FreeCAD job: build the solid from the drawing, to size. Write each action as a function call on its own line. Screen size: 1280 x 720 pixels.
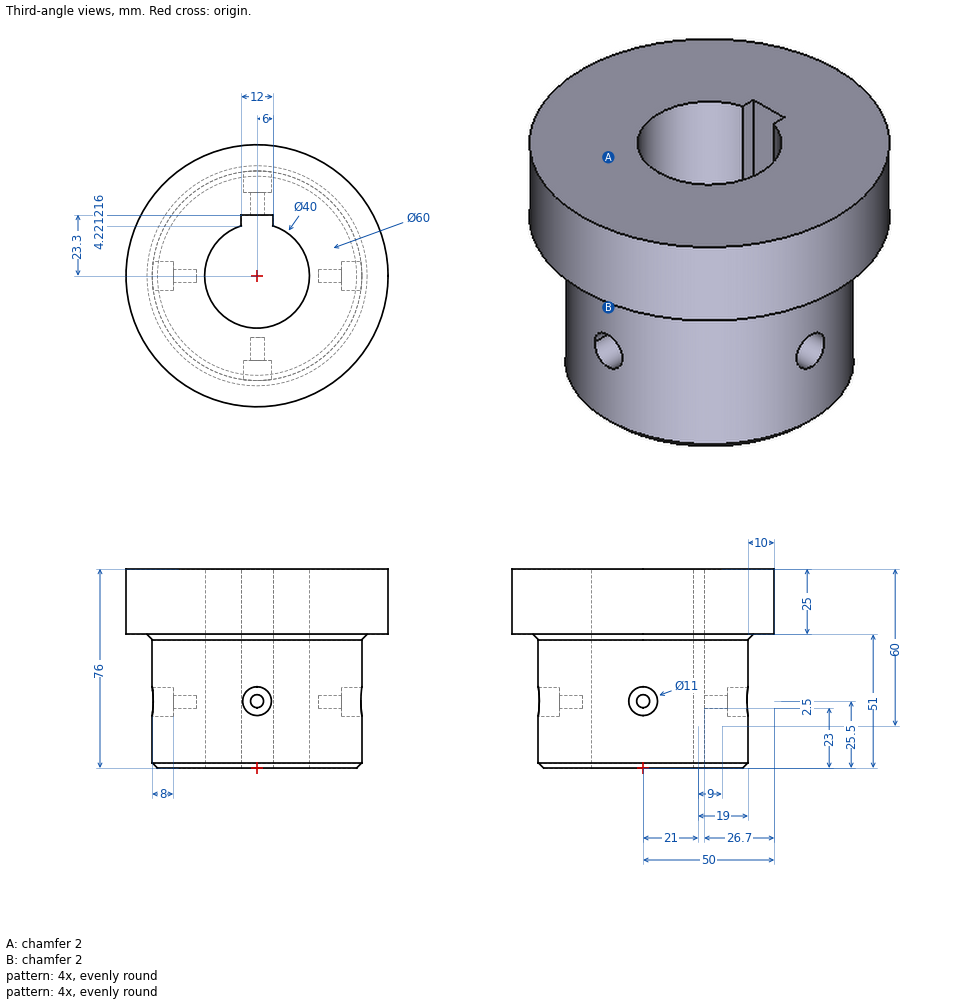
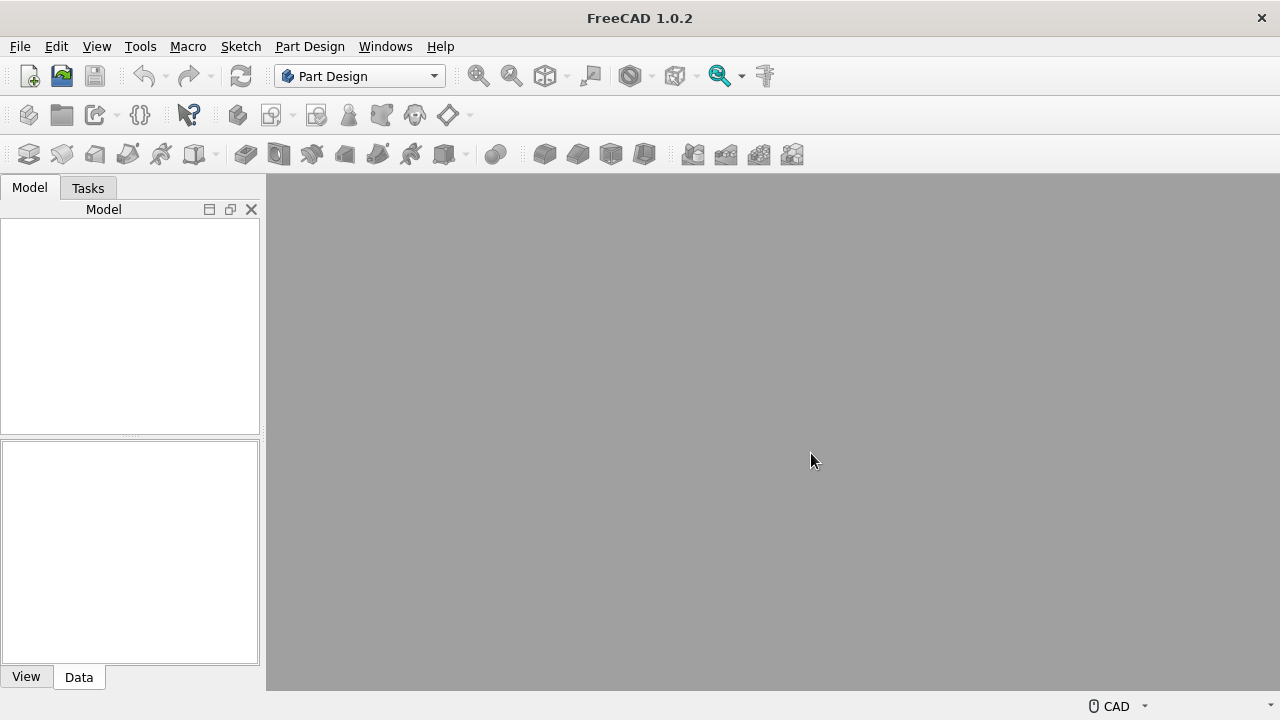
key(ctrl+n)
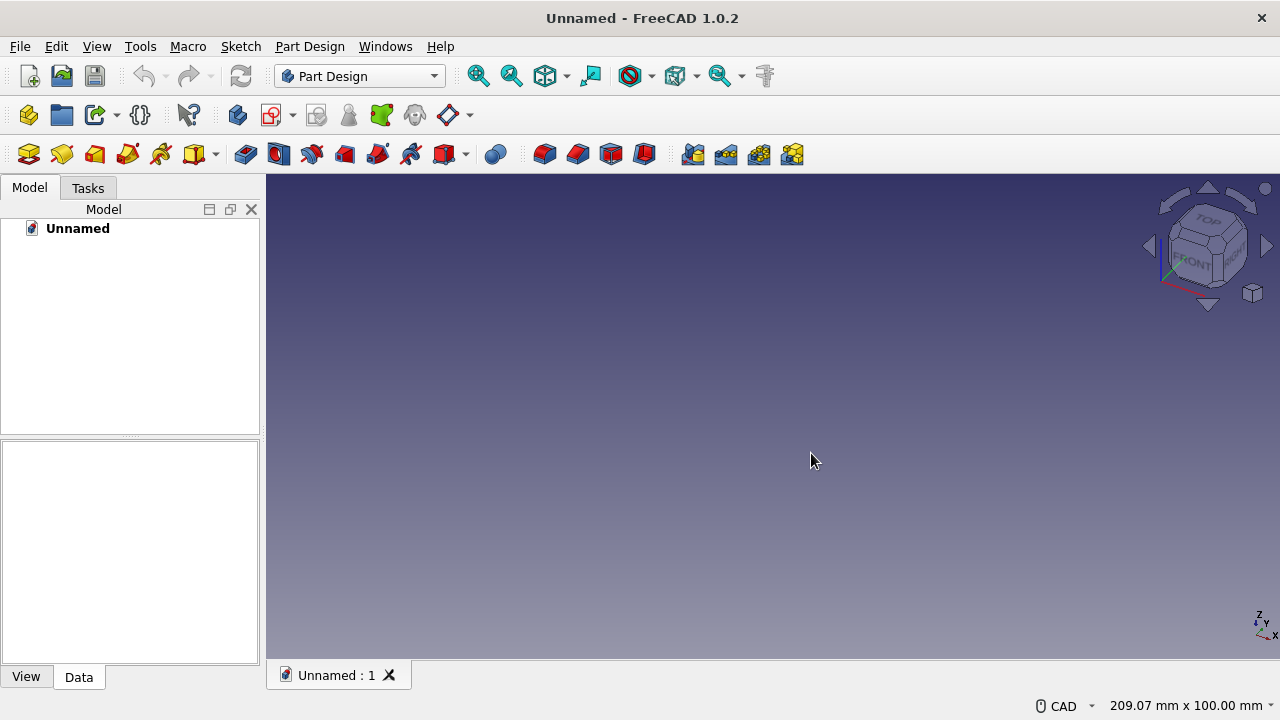
click(270, 116)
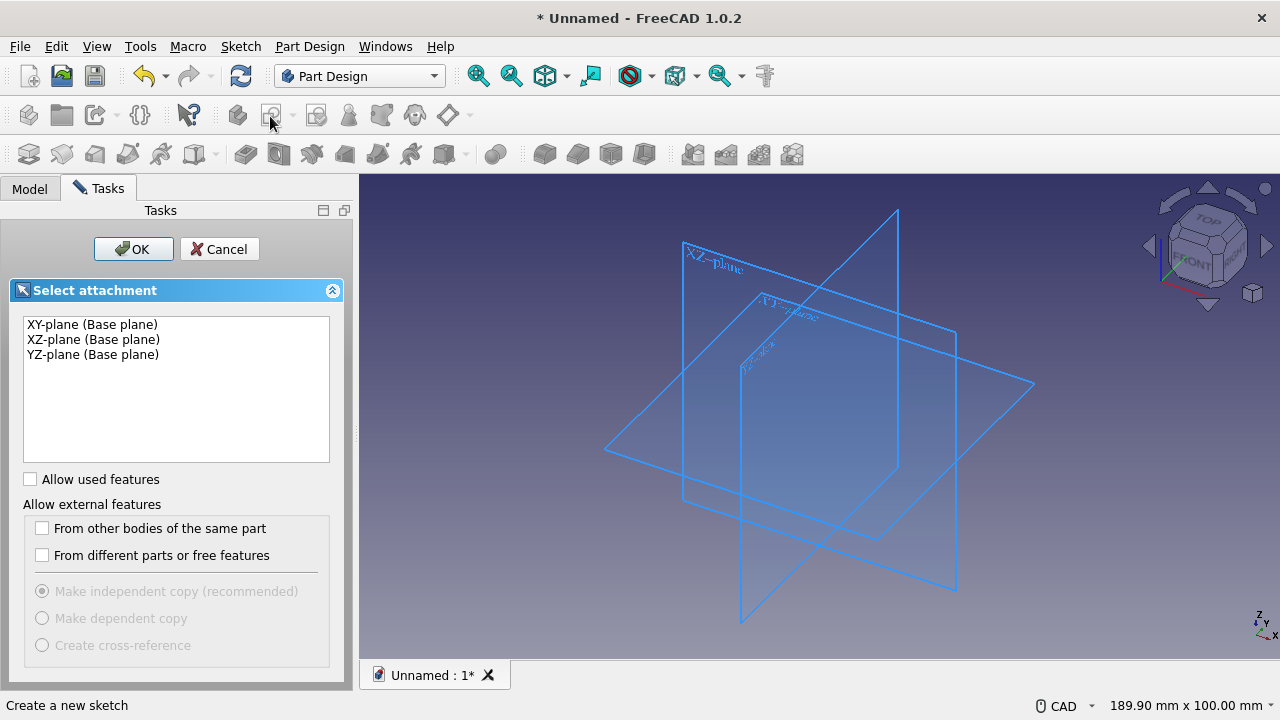
click(84, 354)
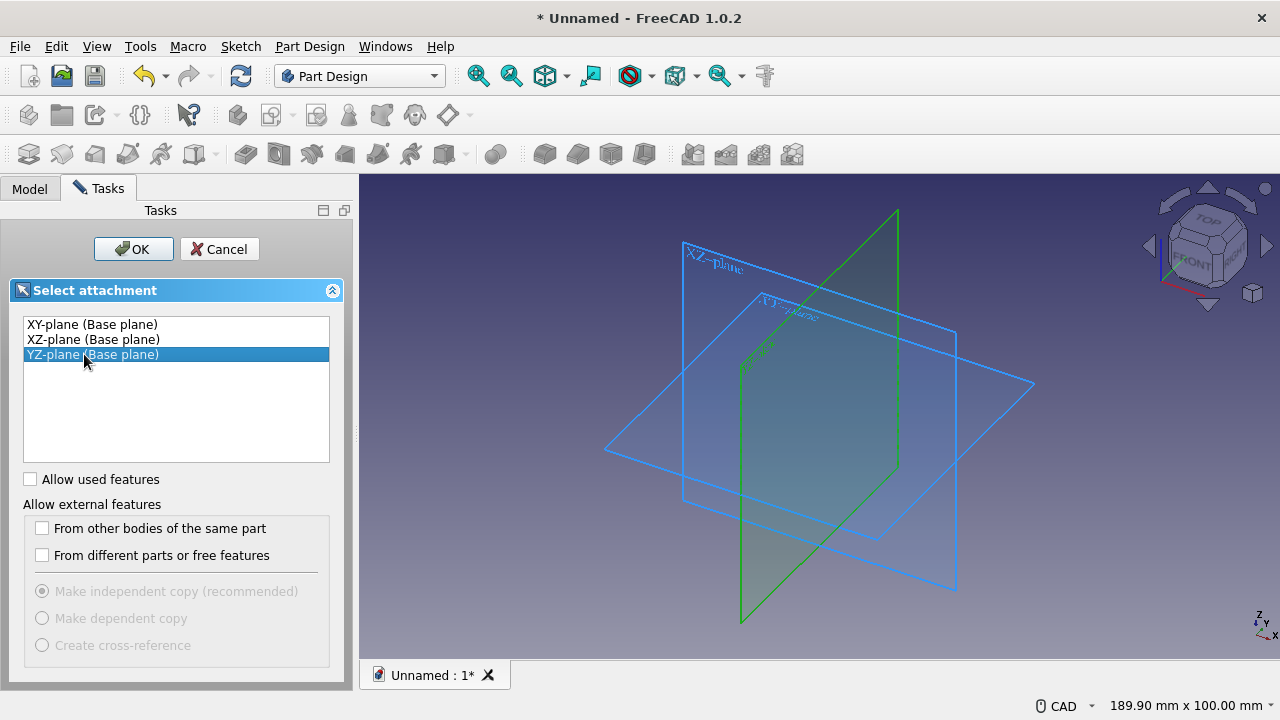
click(134, 249)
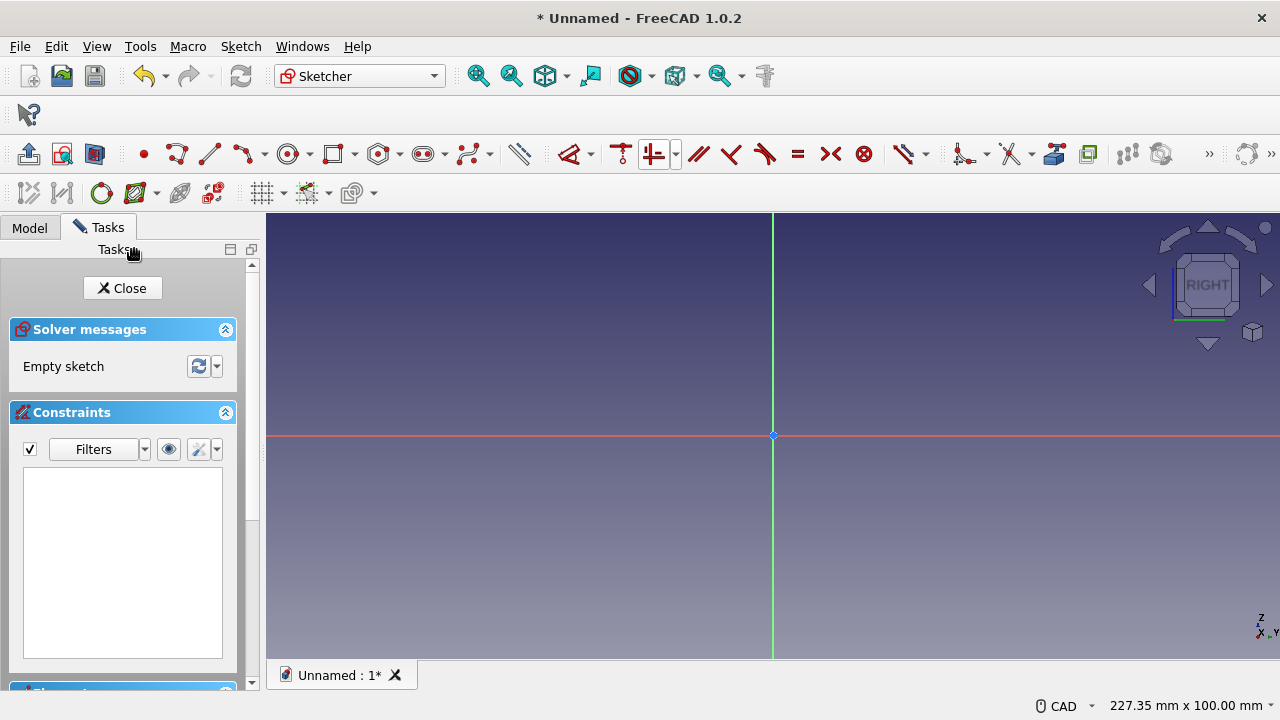
scroll(339, 631, down, 2)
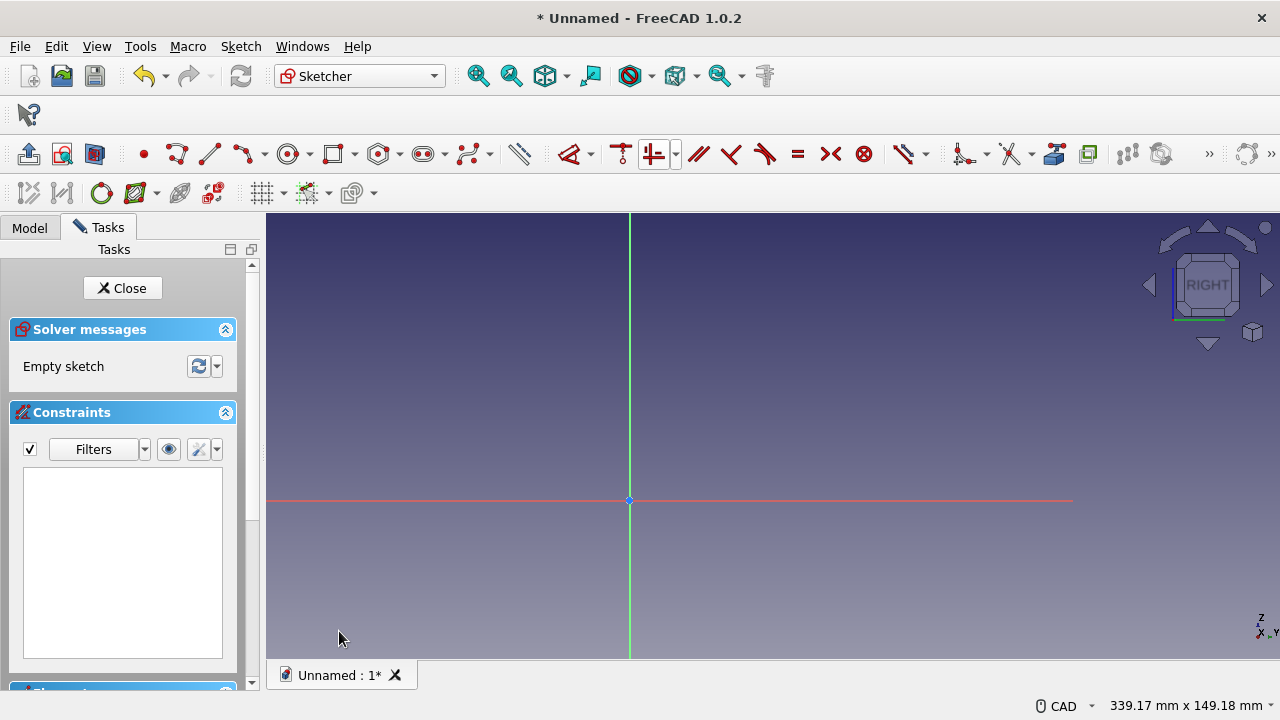
key(g)
key(m)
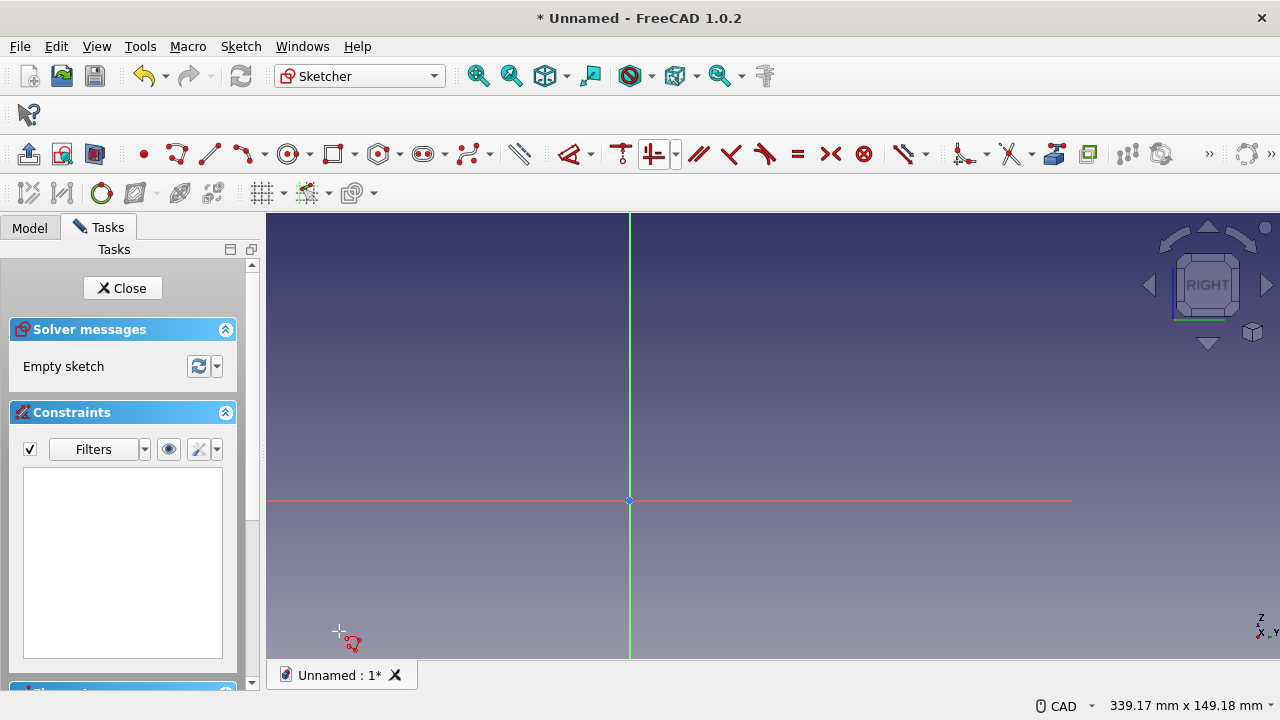
click(693, 501)
click(750, 492)
click(750, 348)
click(779, 348)
click(779, 273)
click(720, 273)
click(720, 453)
click(693, 453)
click(693, 501)
key(Escape)
key(Escape)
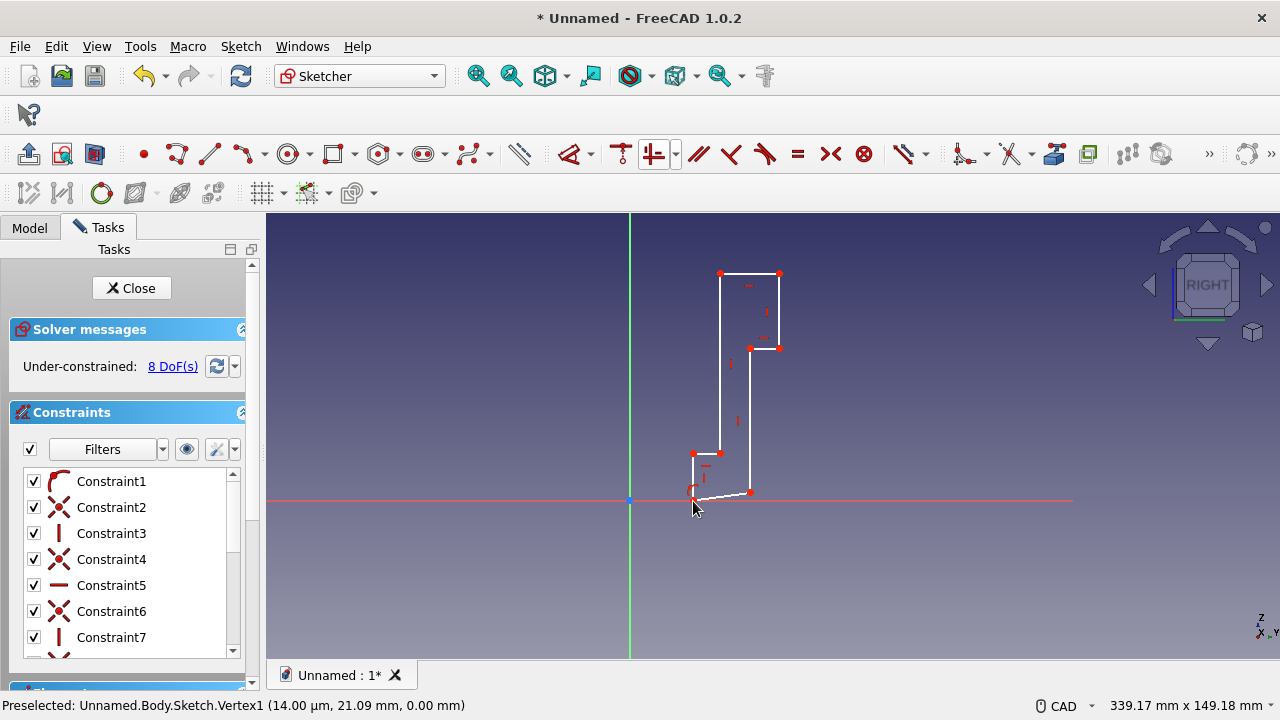
click(710, 498)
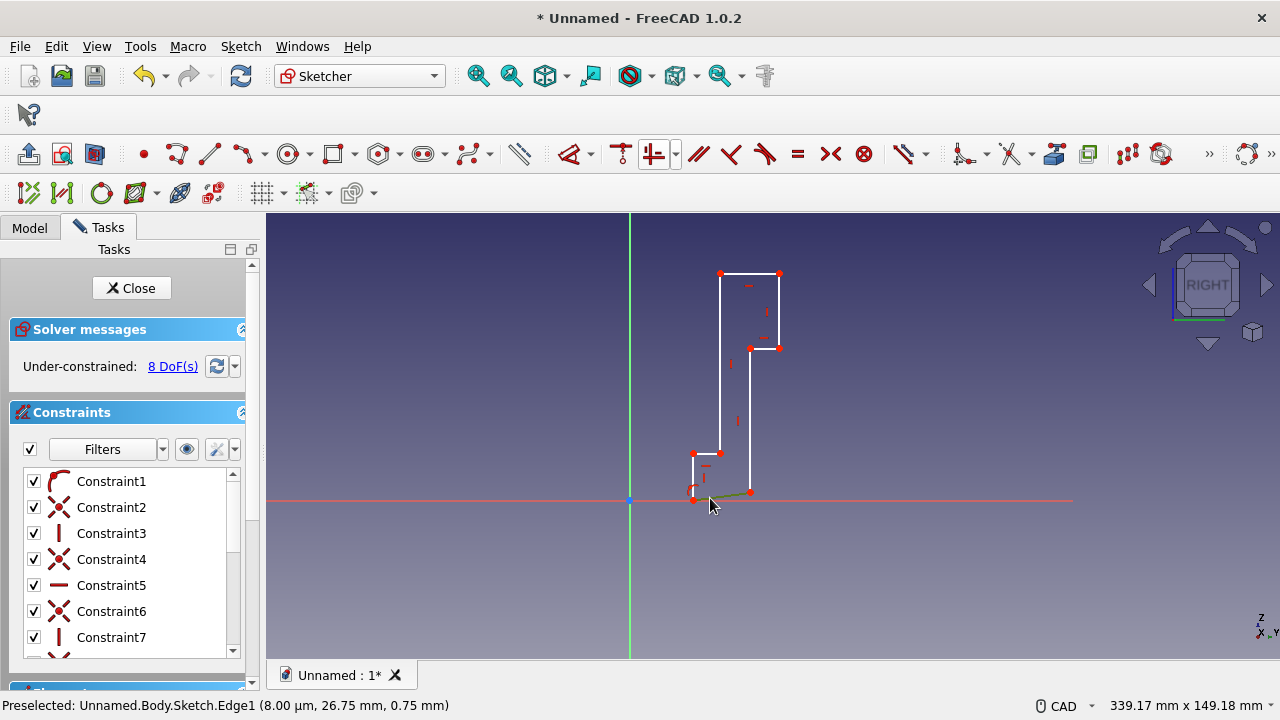
click(676, 154)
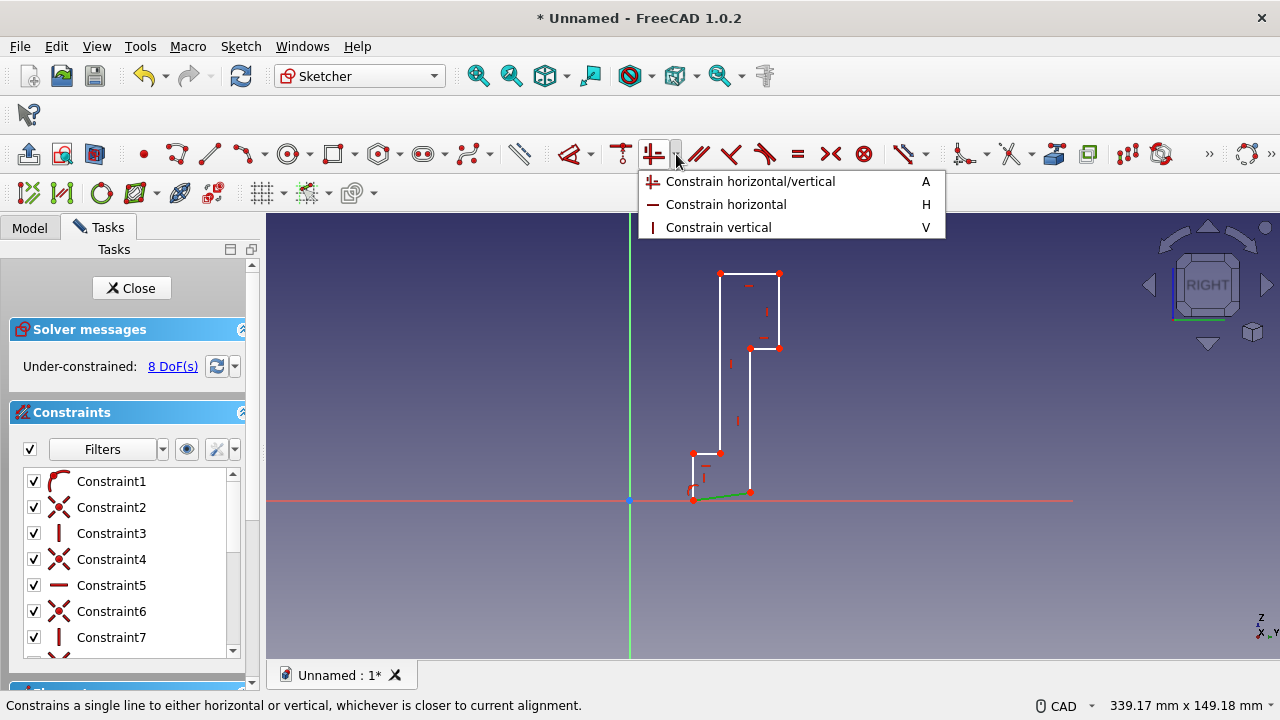
click(792, 204)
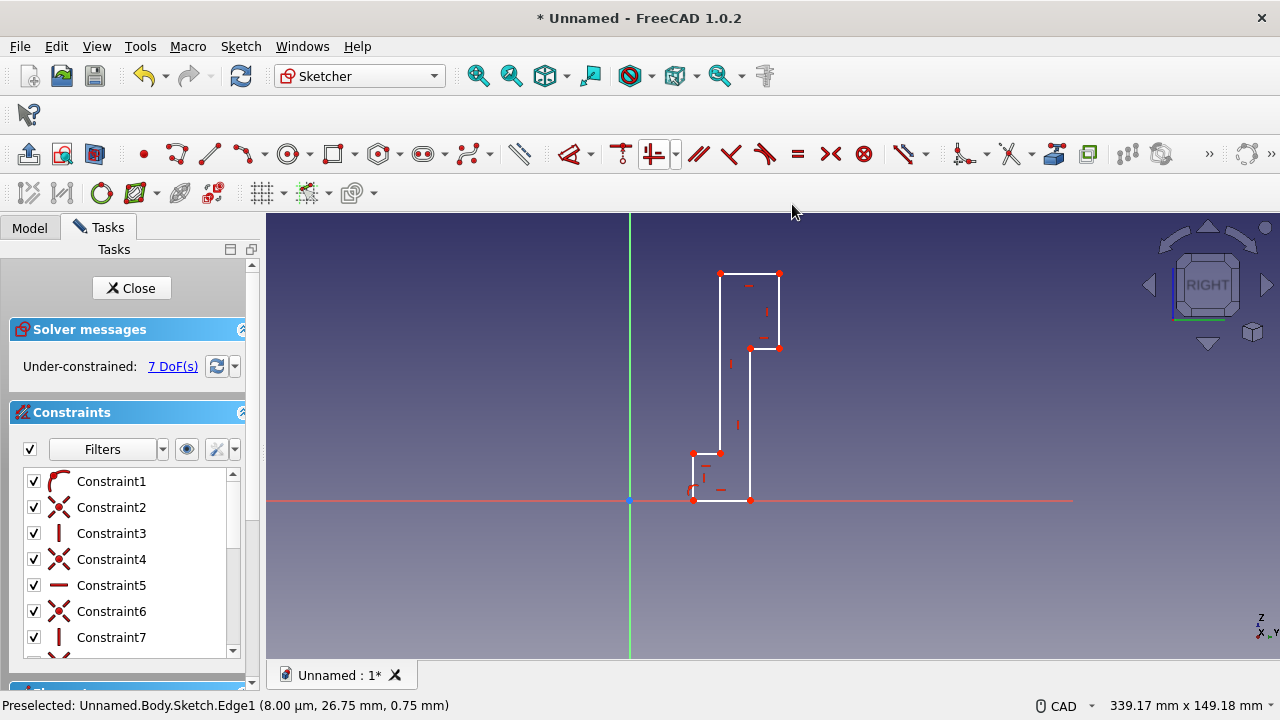
click(568, 154)